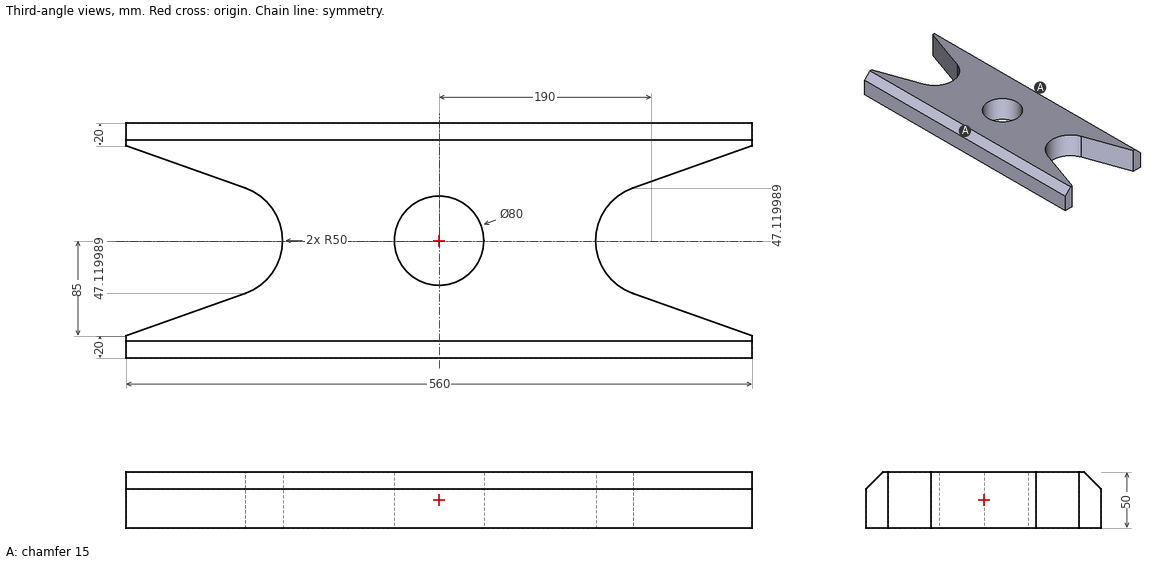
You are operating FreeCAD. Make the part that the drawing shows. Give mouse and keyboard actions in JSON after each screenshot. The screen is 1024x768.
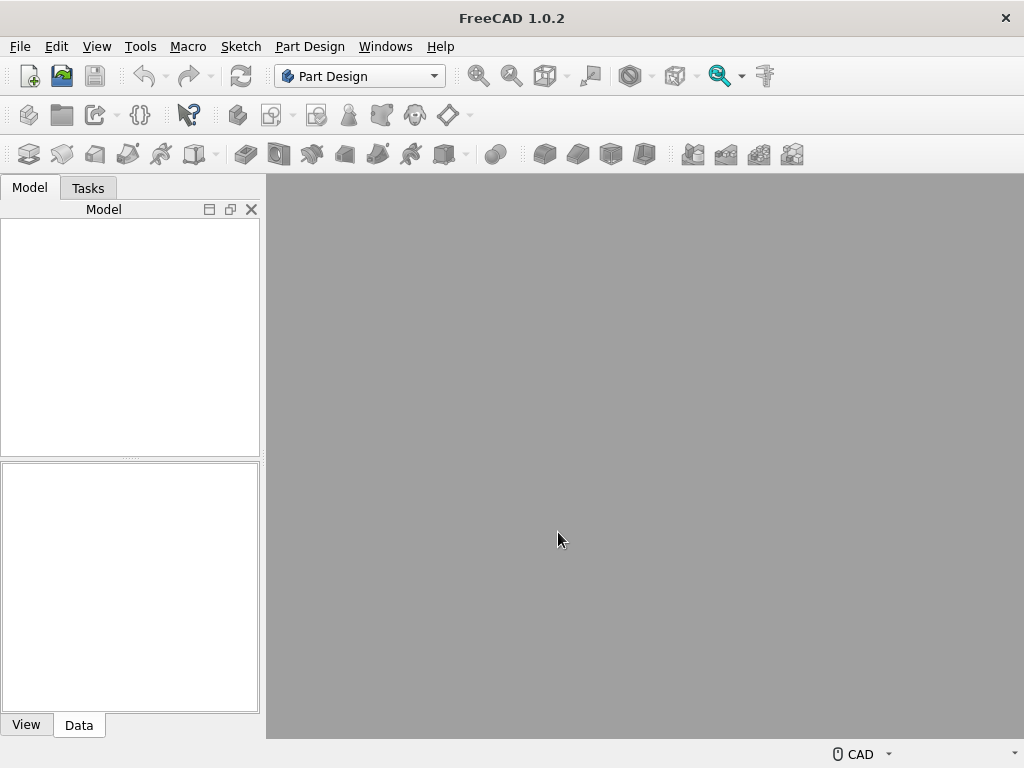
{"action": "key", "text": "ctrl+n"}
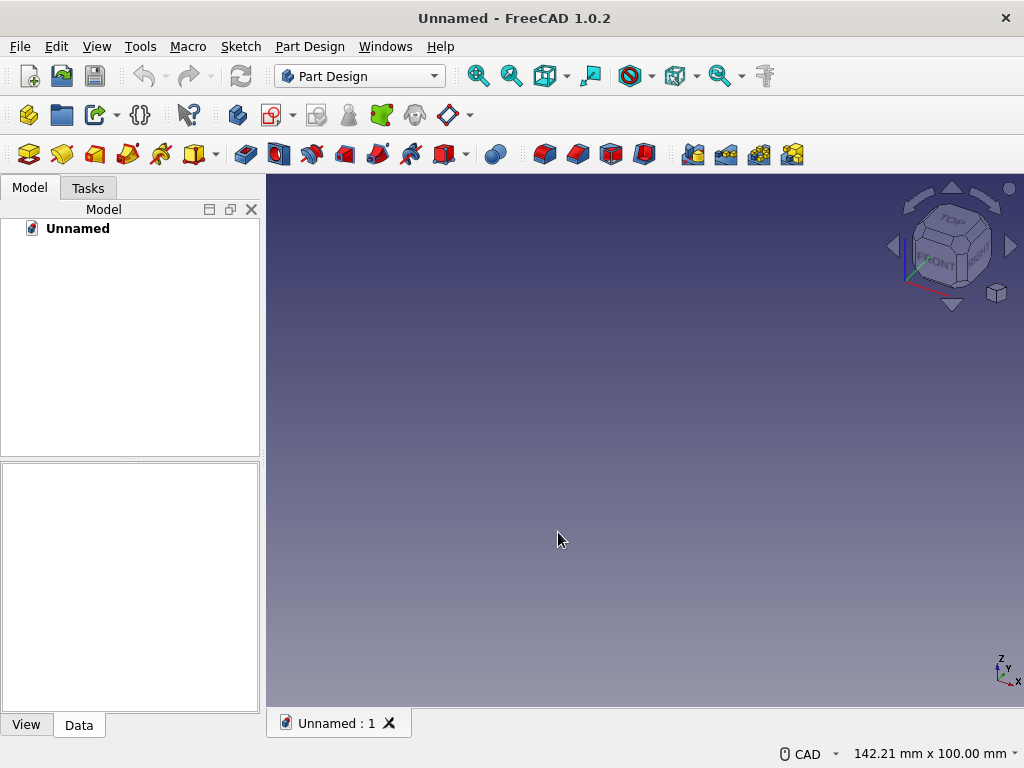
{"action": "left_click", "coordinate": [270, 116]}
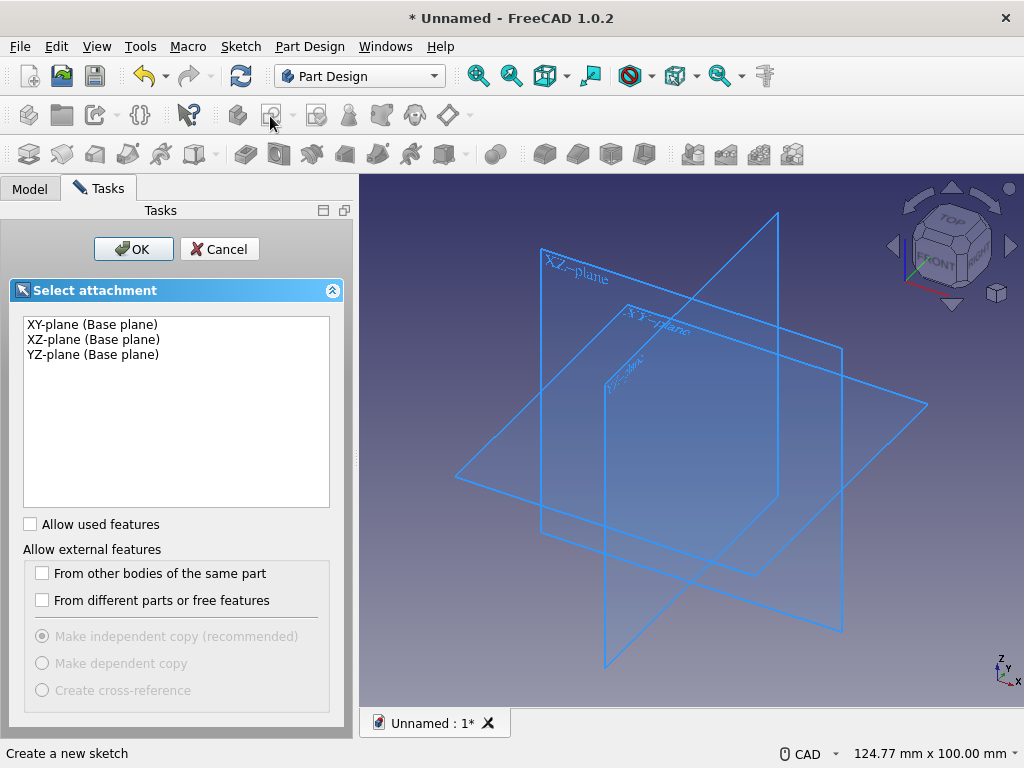
{"action": "left_click", "coordinate": [84, 324]}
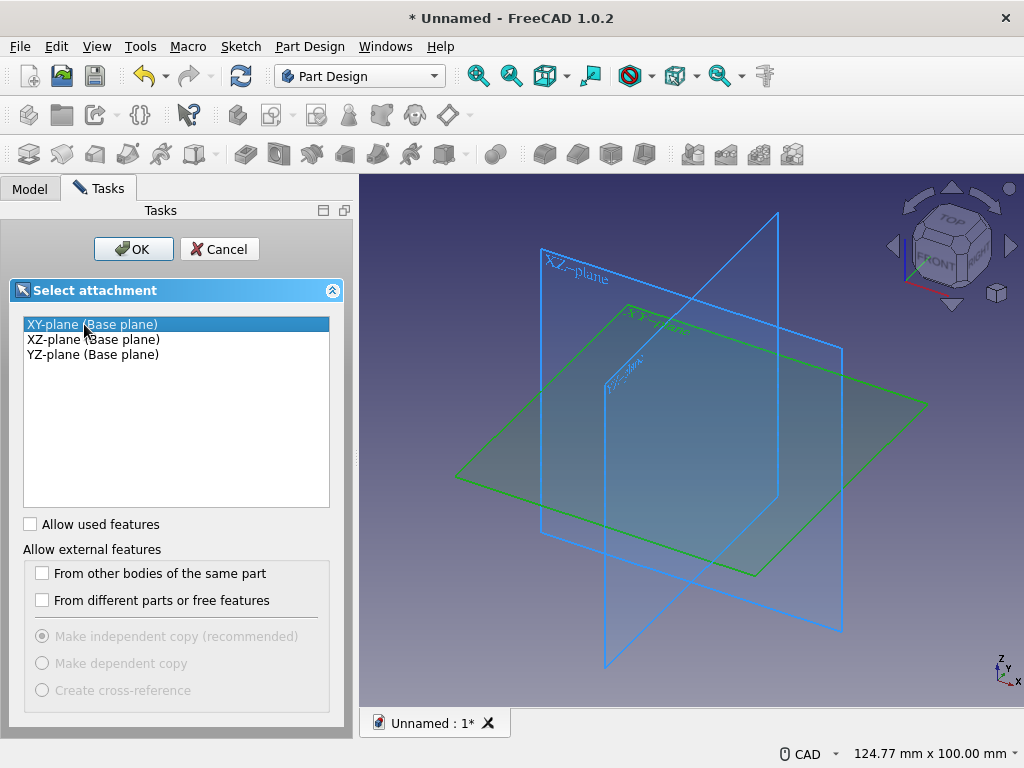
{"action": "left_click", "coordinate": [134, 249]}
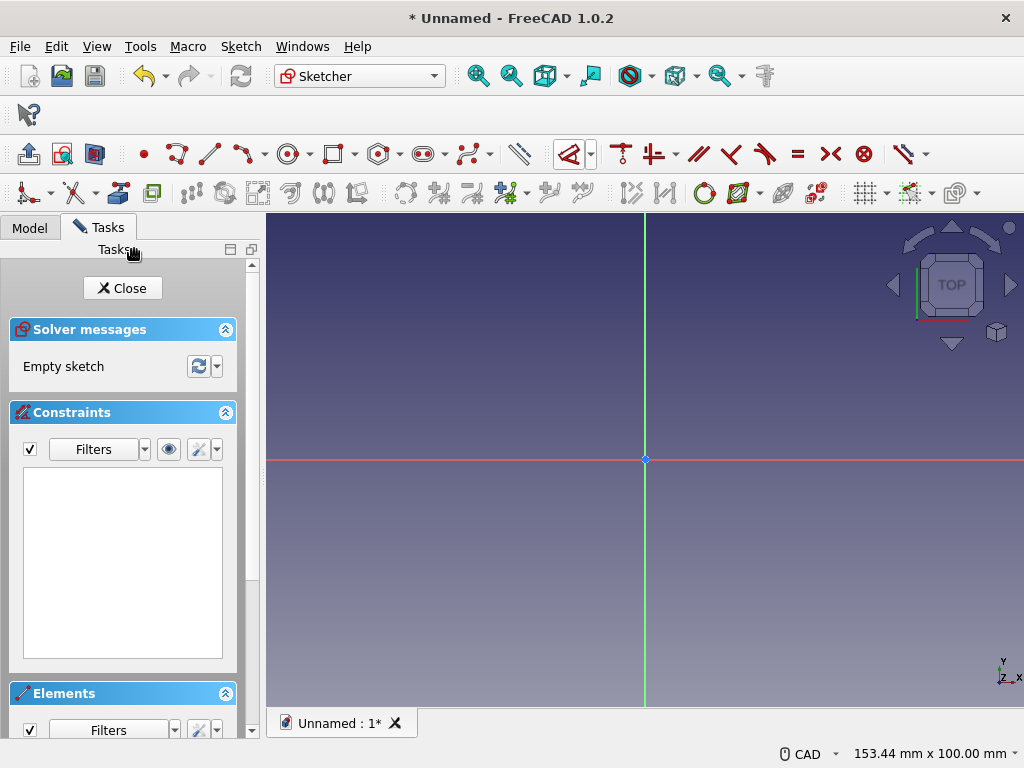
{"action": "scroll", "coordinate": [566, 460], "scroll_direction": "down", "scroll_amount": 10}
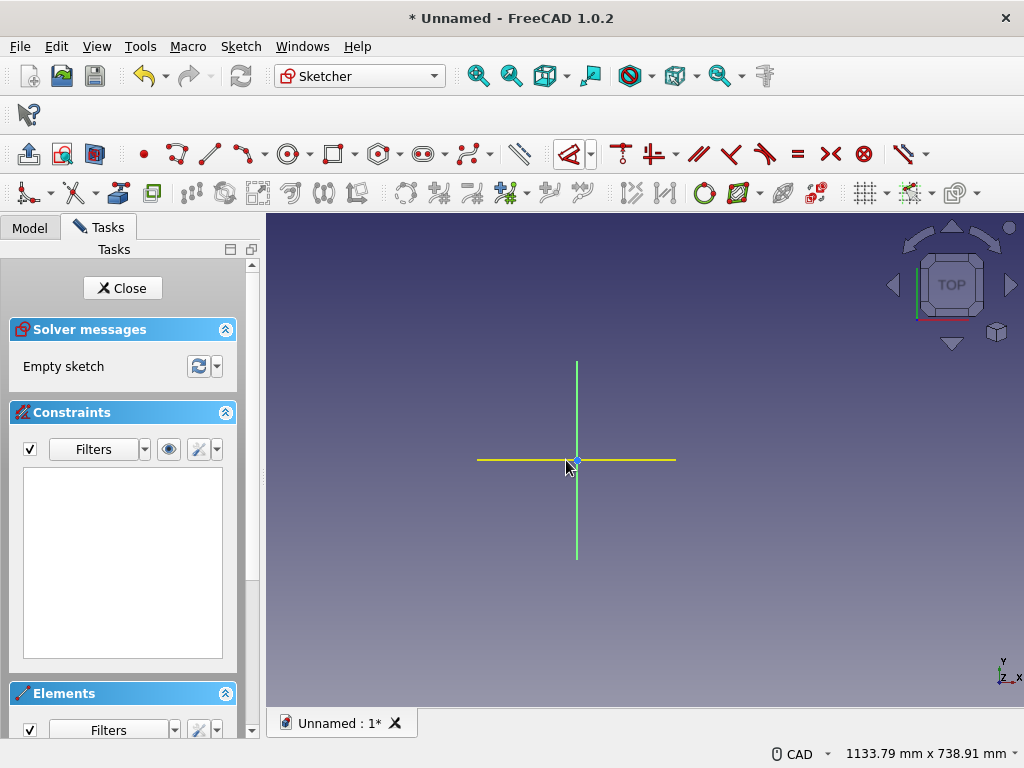
{"action": "key", "text": "g m"}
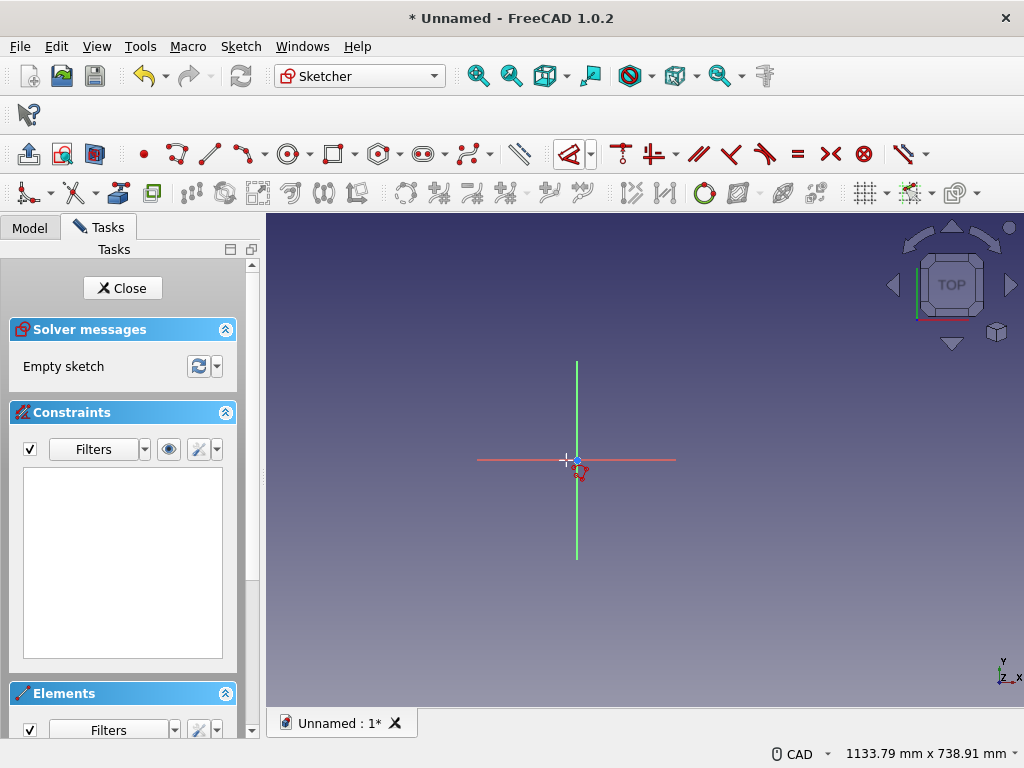
{"action": "left_click", "coordinate": [461, 492]}
{"action": "left_click", "coordinate": [390, 517]}
{"action": "left_click", "coordinate": [390, 531]}
{"action": "left_click", "coordinate": [764, 531]}
{"action": "left_click", "coordinate": [764, 517]}
{"action": "left_click", "coordinate": [693, 492]}
{"action": "right_click", "coordinate": [693, 492]}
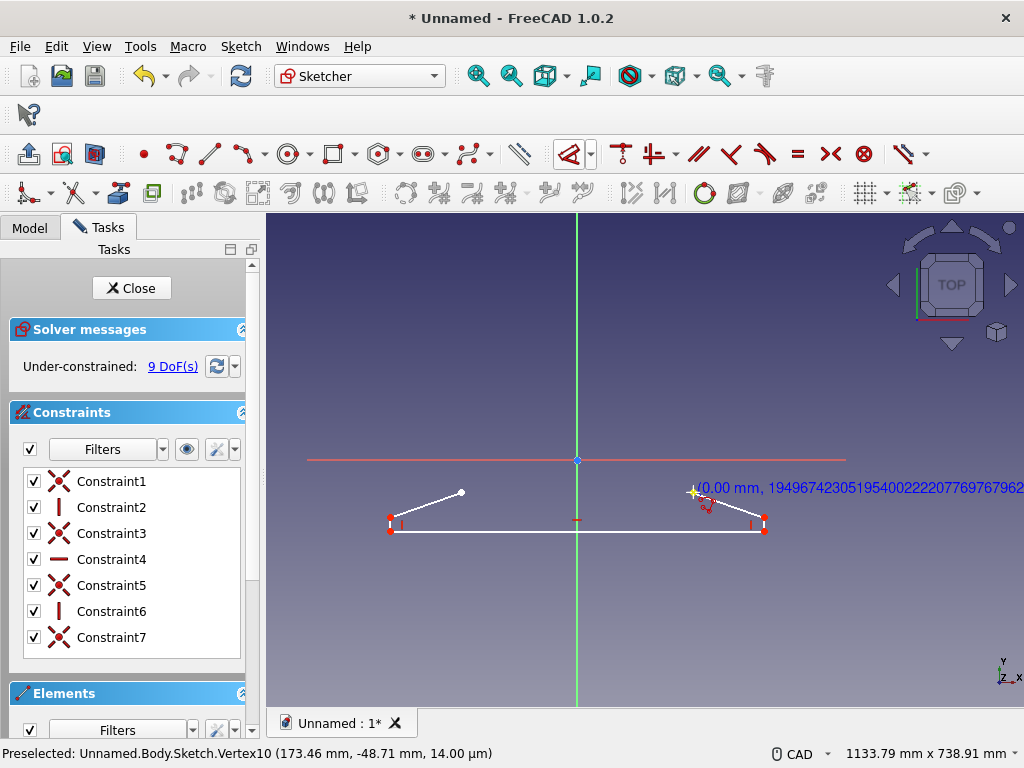
{"action": "left_click", "coordinate": [693, 429]}
{"action": "left_click", "coordinate": [764, 404]}
{"action": "left_click", "coordinate": [764, 390]}
{"action": "left_click", "coordinate": [390, 390]}
{"action": "left_click", "coordinate": [390, 404]}
{"action": "left_click", "coordinate": [461, 429]}
{"action": "right_click", "coordinate": [461, 429]}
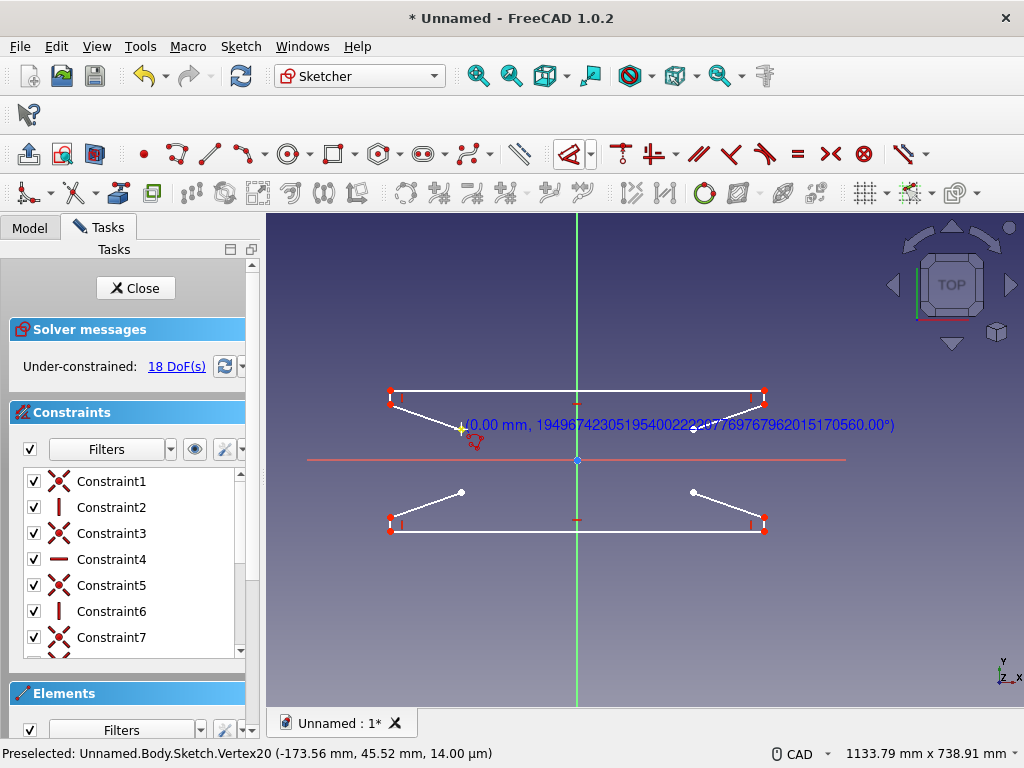
{"action": "key", "text": "g 3 a"}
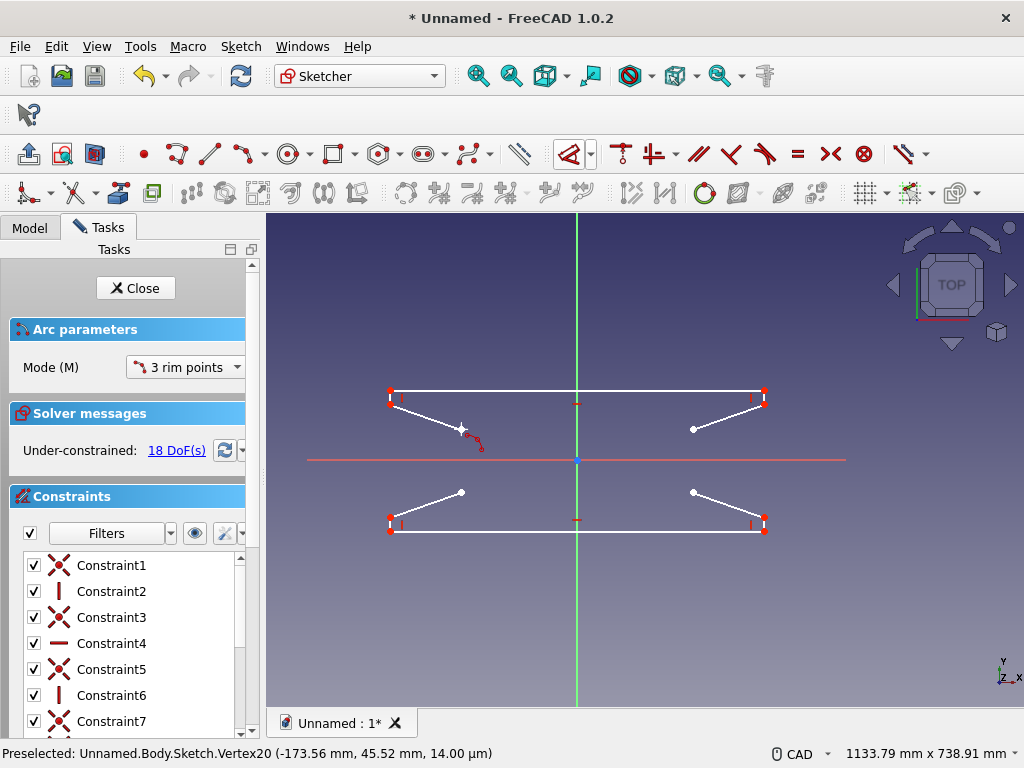
{"action": "left_click", "coordinate": [693, 493]}
{"action": "left_click", "coordinate": [693, 430]}
{"action": "left_click", "coordinate": [675, 445]}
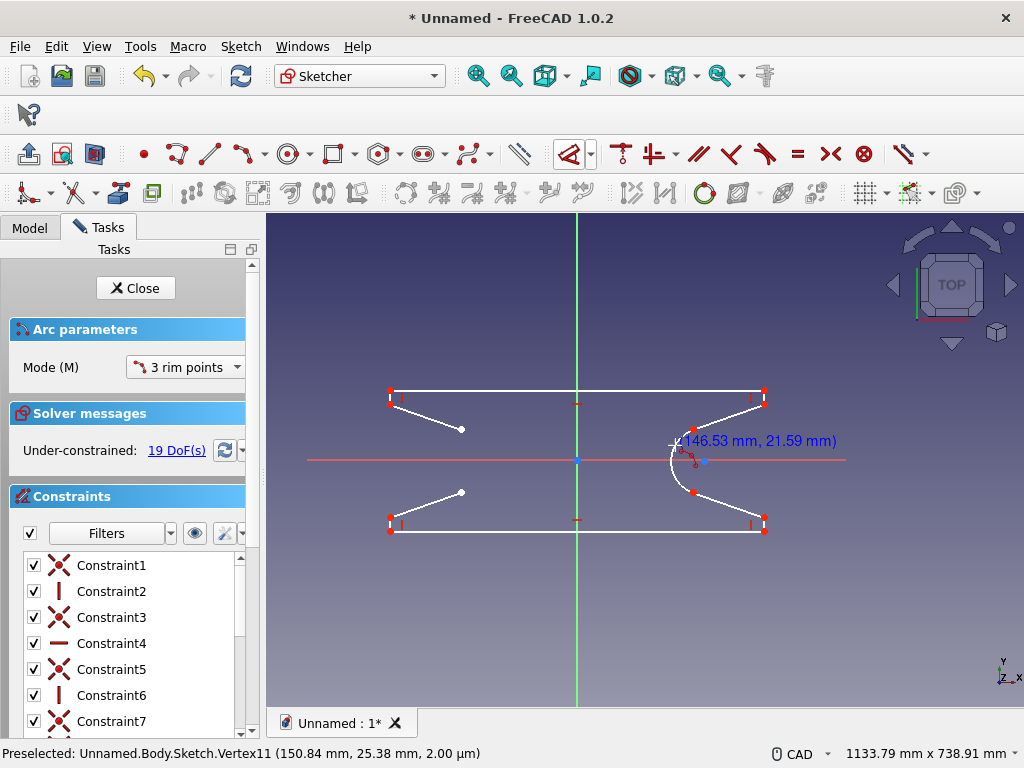
{"action": "left_click", "coordinate": [461, 430]}
{"action": "left_click", "coordinate": [461, 493]}
{"action": "left_click", "coordinate": [479, 476]}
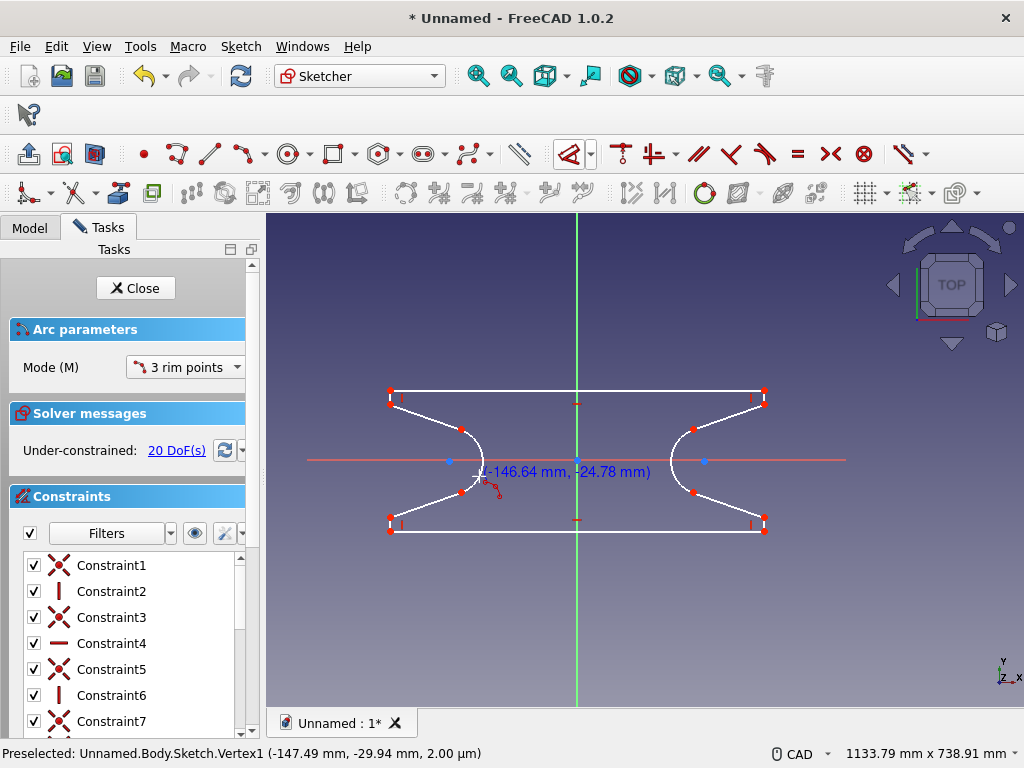
{"action": "key", "text": "g c"}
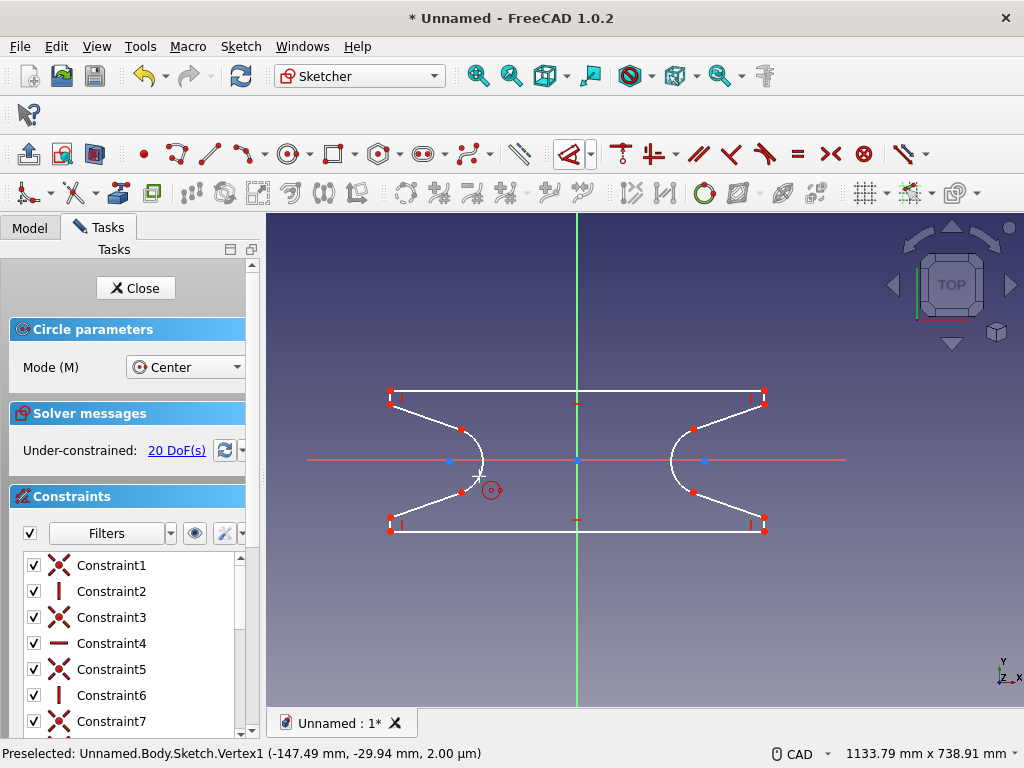
{"action": "left_click", "coordinate": [577, 460]}
{"action": "mouse_move", "coordinate": [596, 442]}